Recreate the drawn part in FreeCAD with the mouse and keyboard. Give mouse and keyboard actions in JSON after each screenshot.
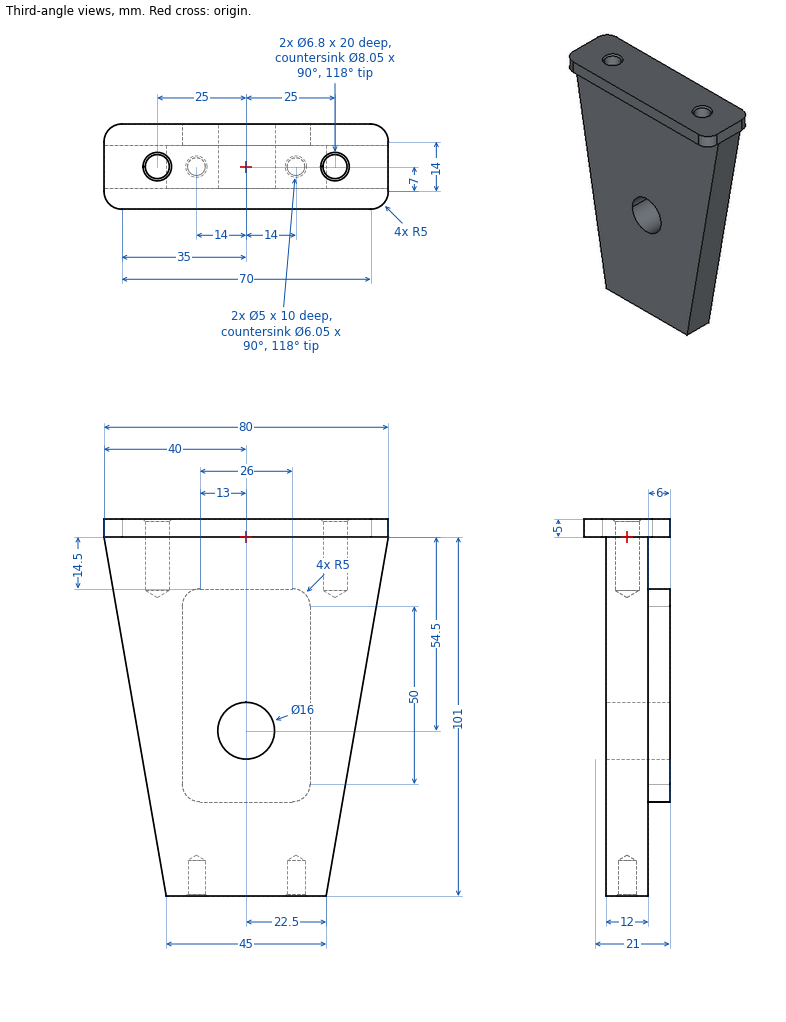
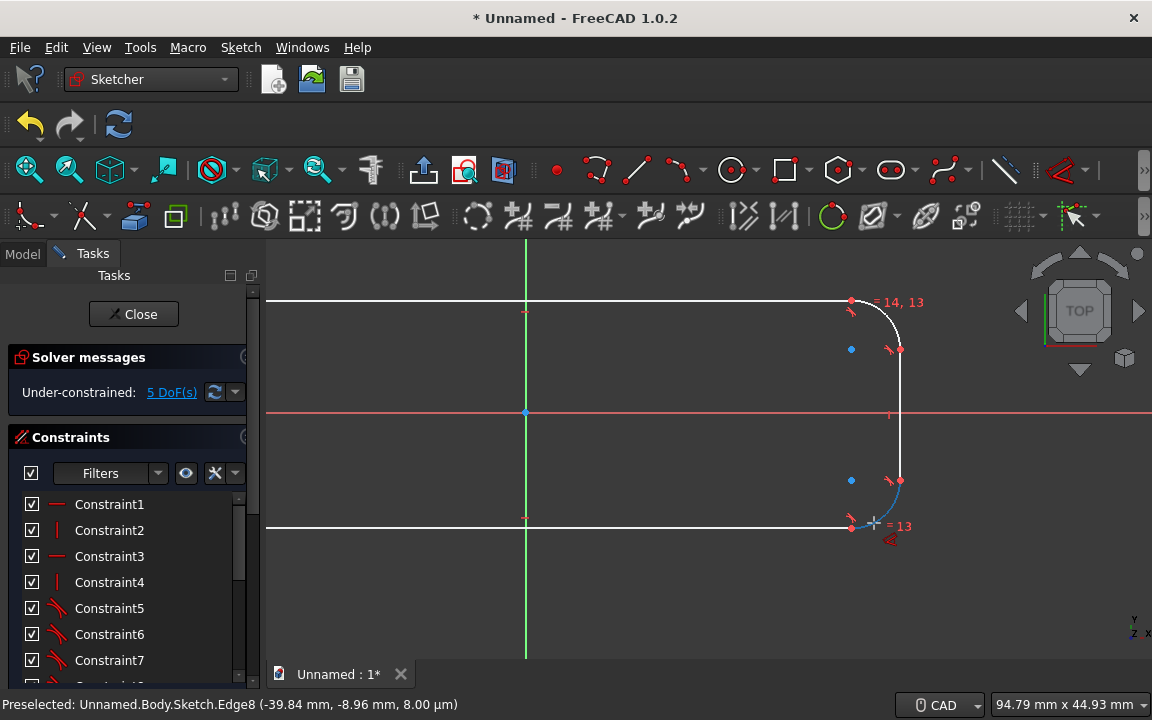
{"action": "left_click", "coordinate": [874, 523]}
{"action": "left_click", "coordinate": [889, 551]}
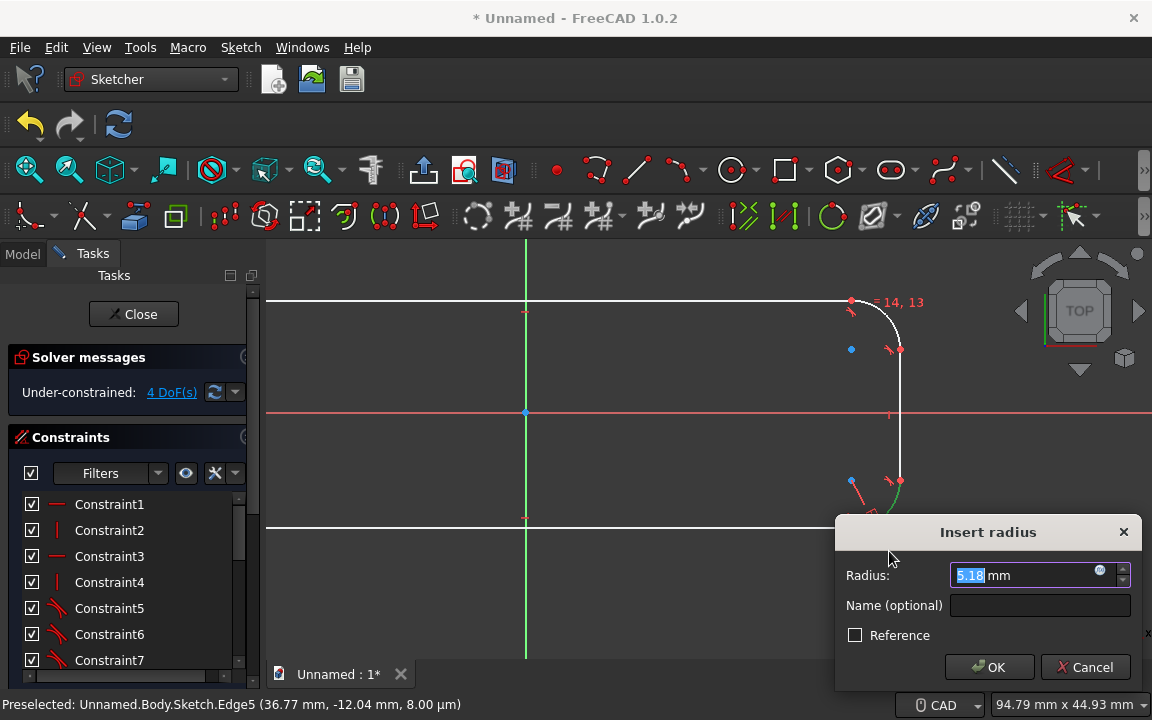
{"action": "type", "text": "5"}
{"action": "key", "text": "Return"}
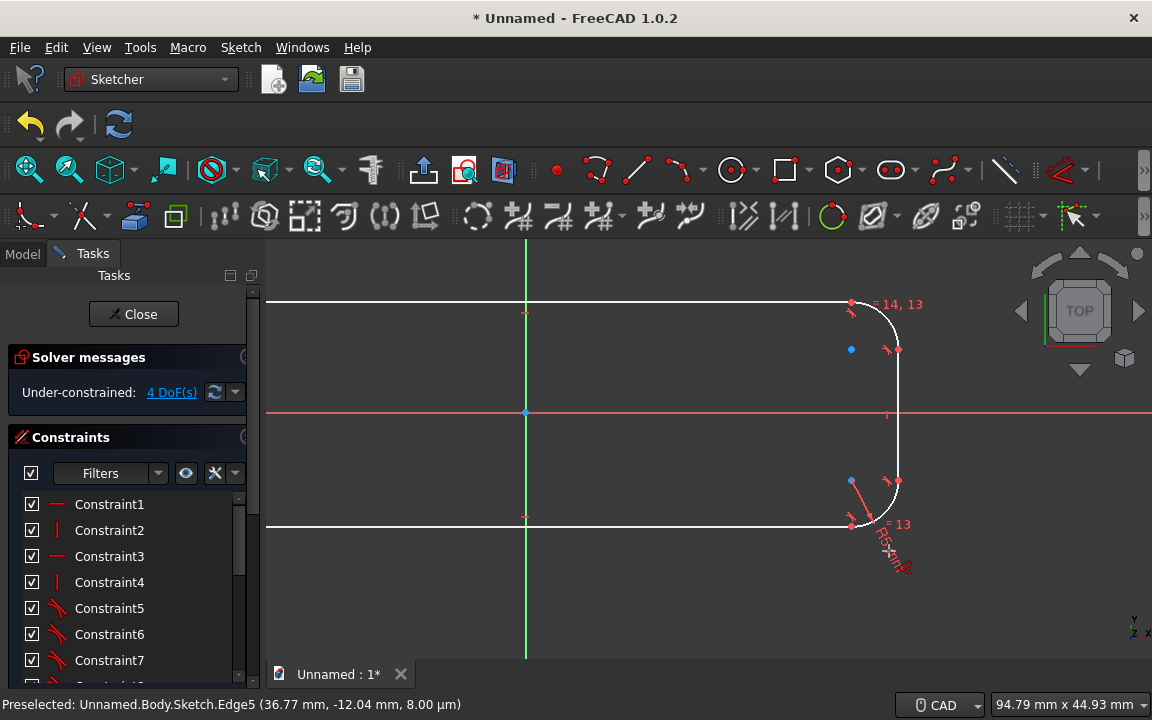
{"action": "left_click", "coordinate": [394, 527]}
{"action": "left_click", "coordinate": [573, 561]}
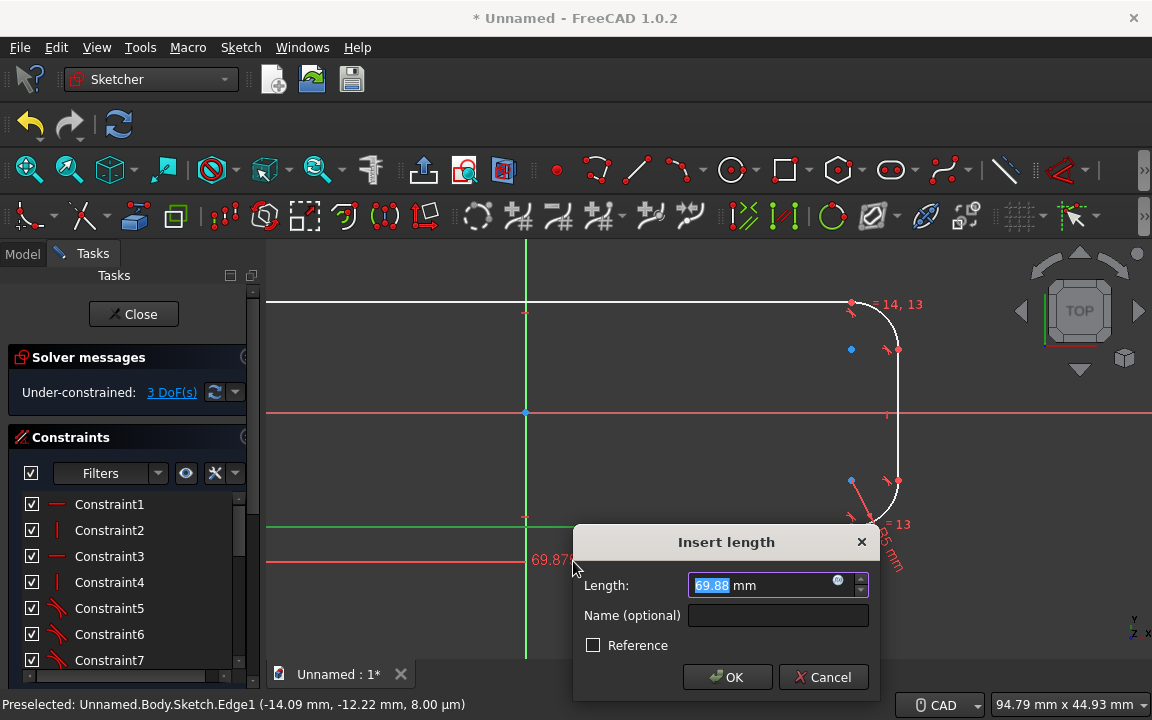
{"action": "type", "text": "70"}
{"action": "key", "text": "Return"}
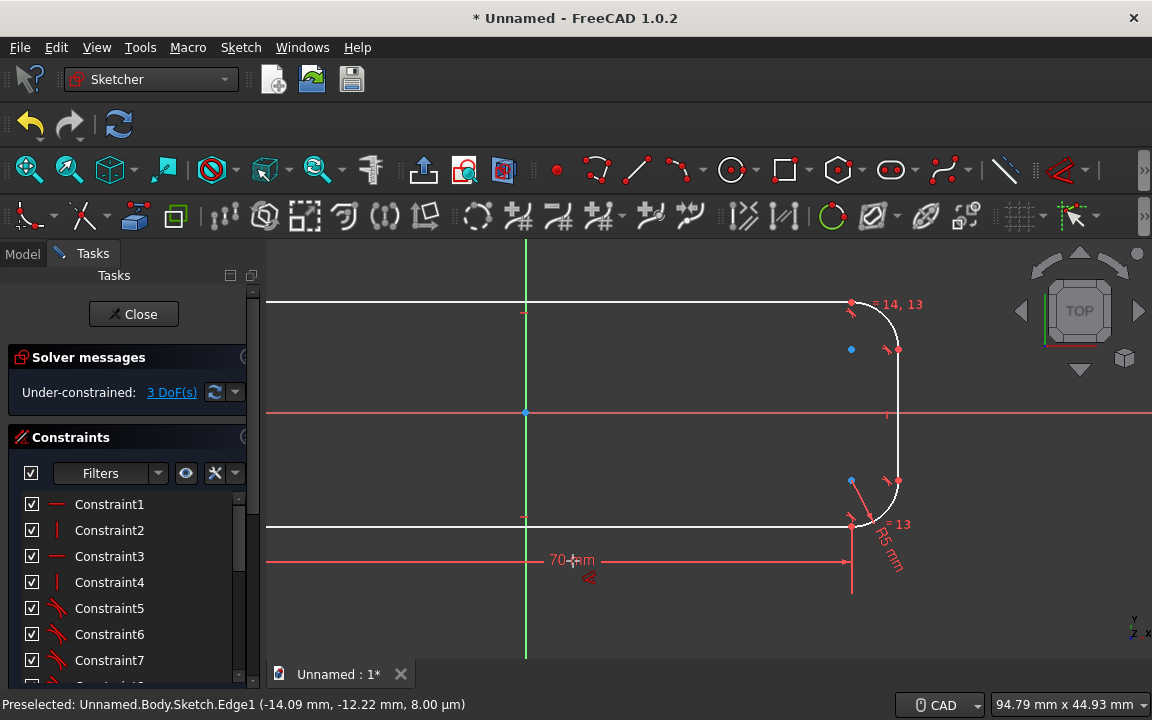
{"action": "left_click", "coordinate": [898, 441]}
{"action": "left_click", "coordinate": [932, 384]}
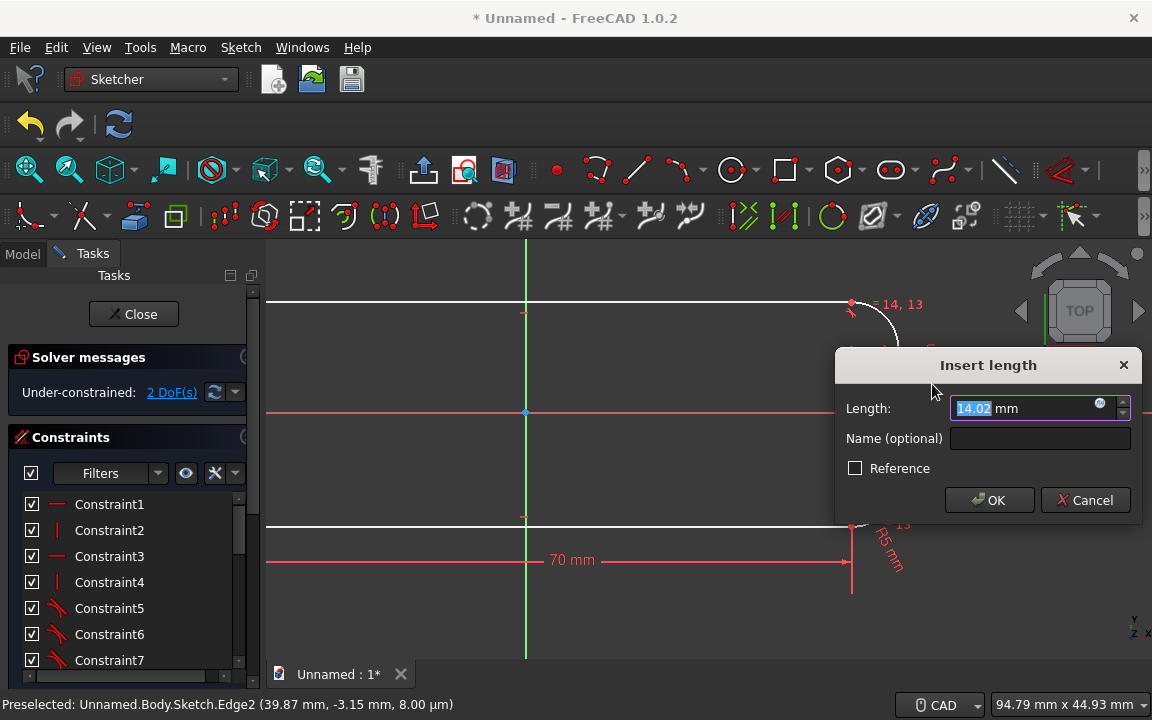
{"action": "type", "text": "14"}
{"action": "key", "text": "Return"}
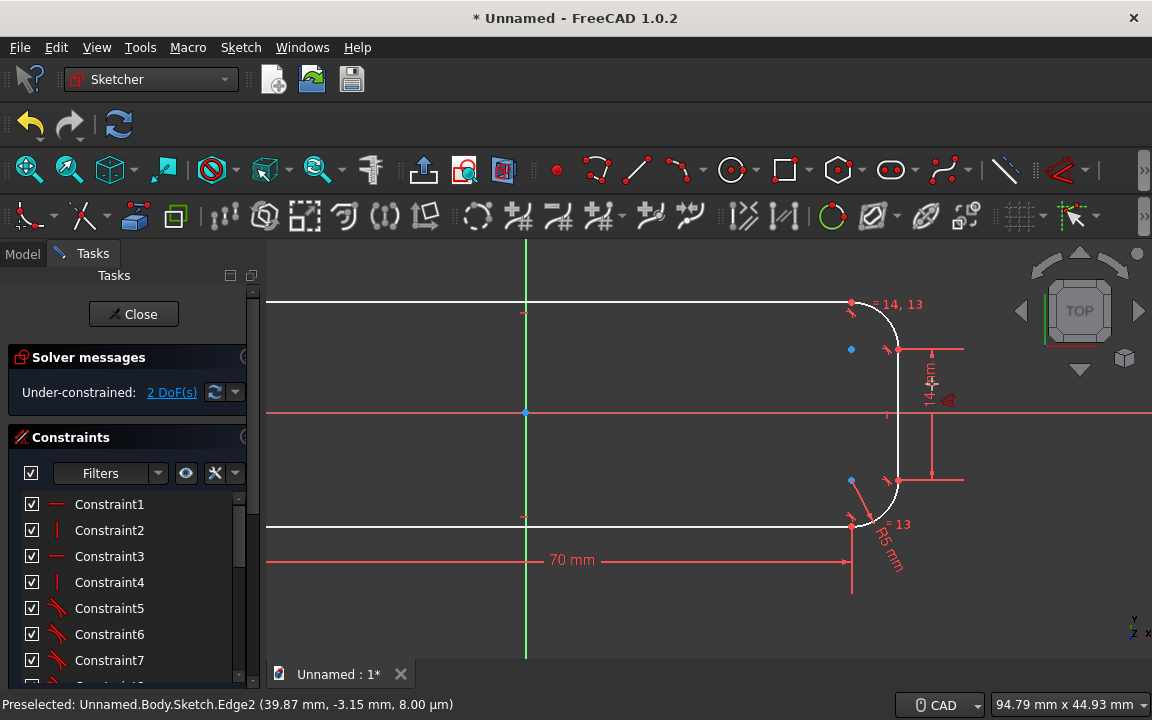
{"action": "left_click", "coordinate": [898, 480]}
{"action": "left_click", "coordinate": [932, 446]}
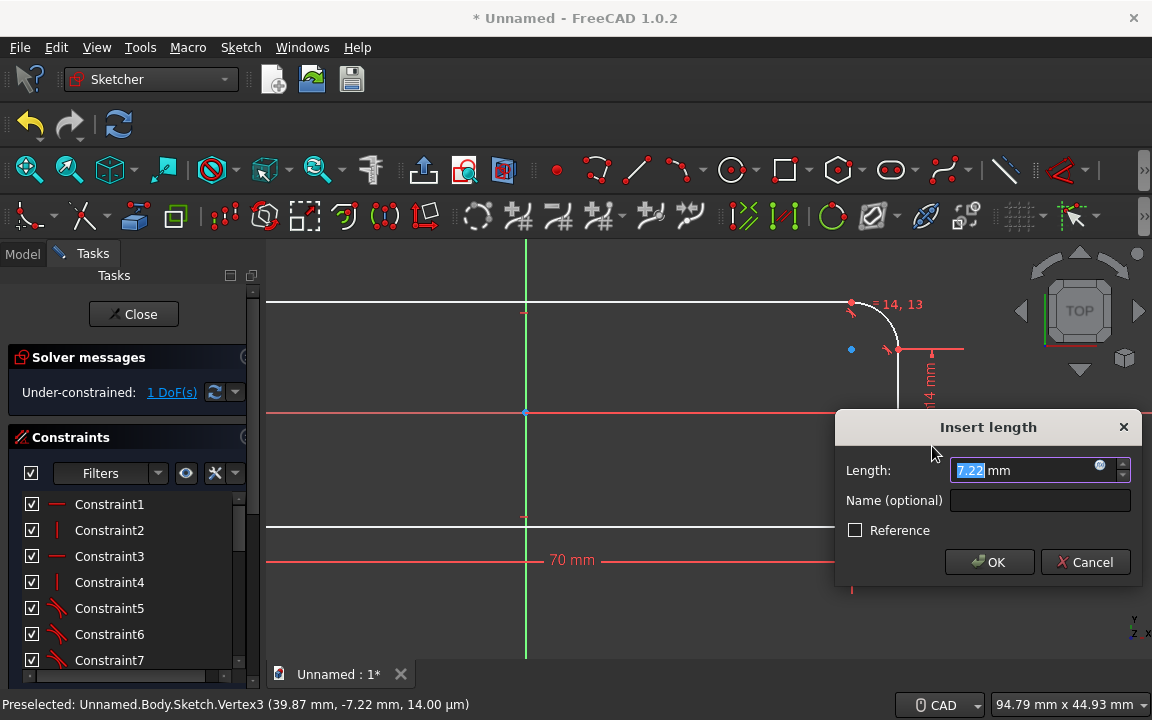
{"action": "type", "text": "7"}
{"action": "key", "text": "Return"}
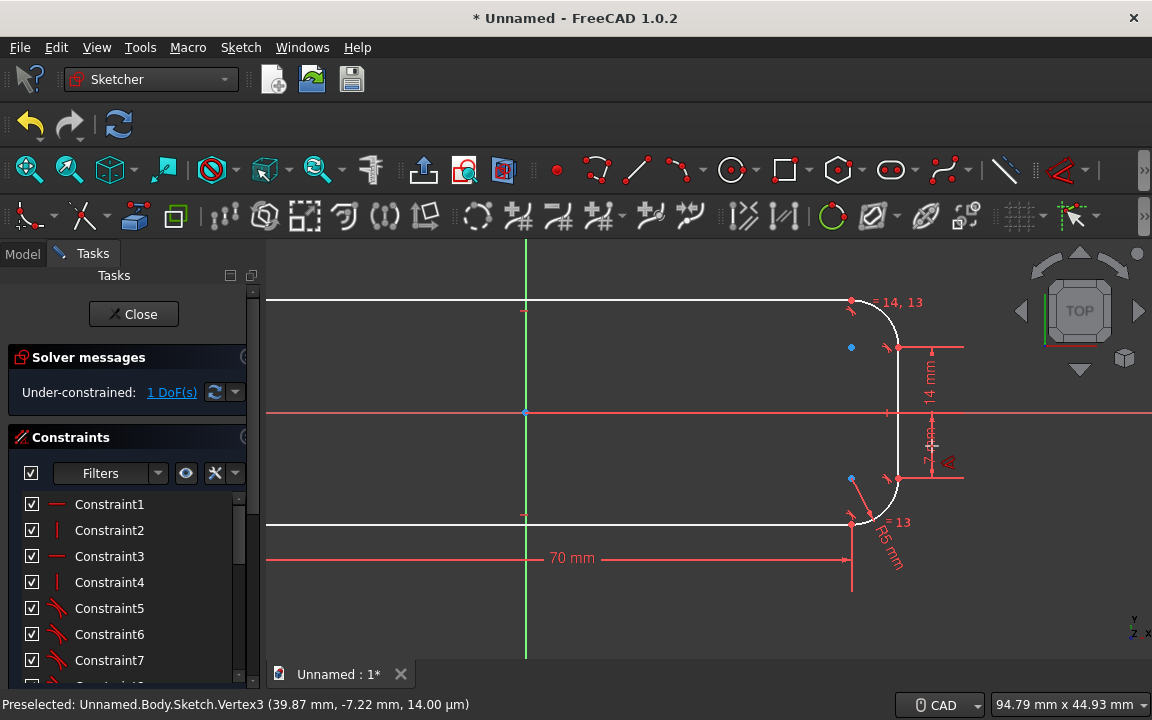
{"action": "scroll", "coordinate": [874, 523], "scroll_direction": "down", "scroll_amount": 2}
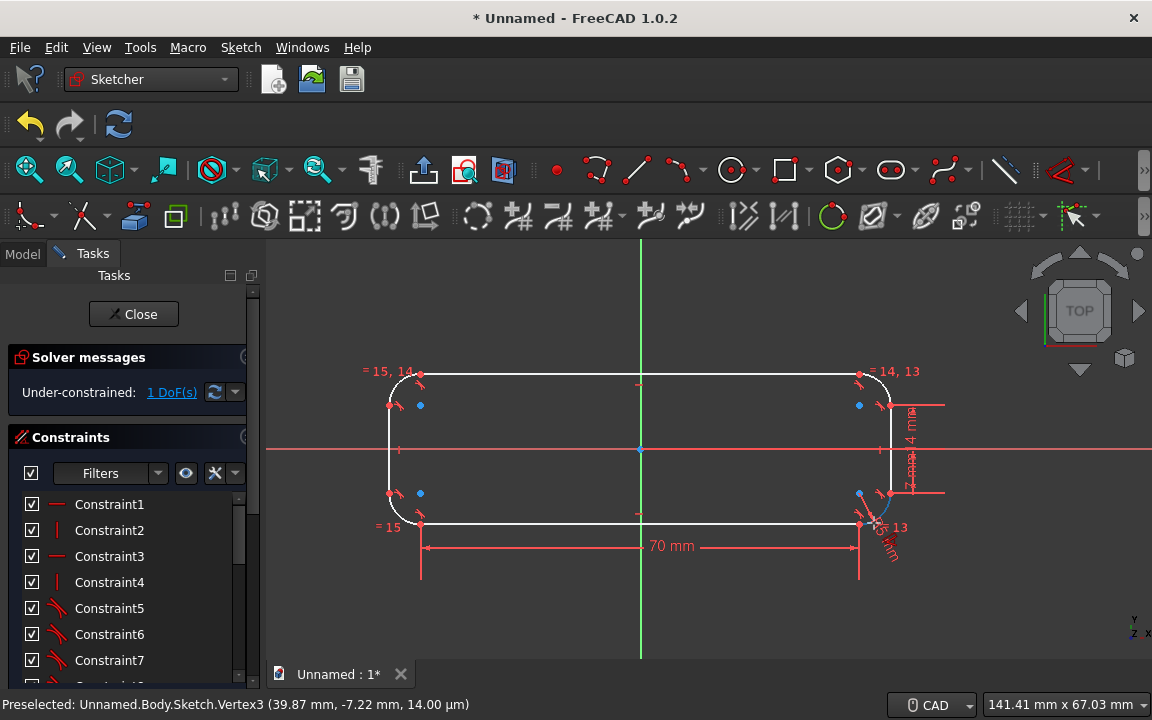
{"action": "left_click", "coordinate": [421, 524]}
{"action": "left_click", "coordinate": [531, 558]}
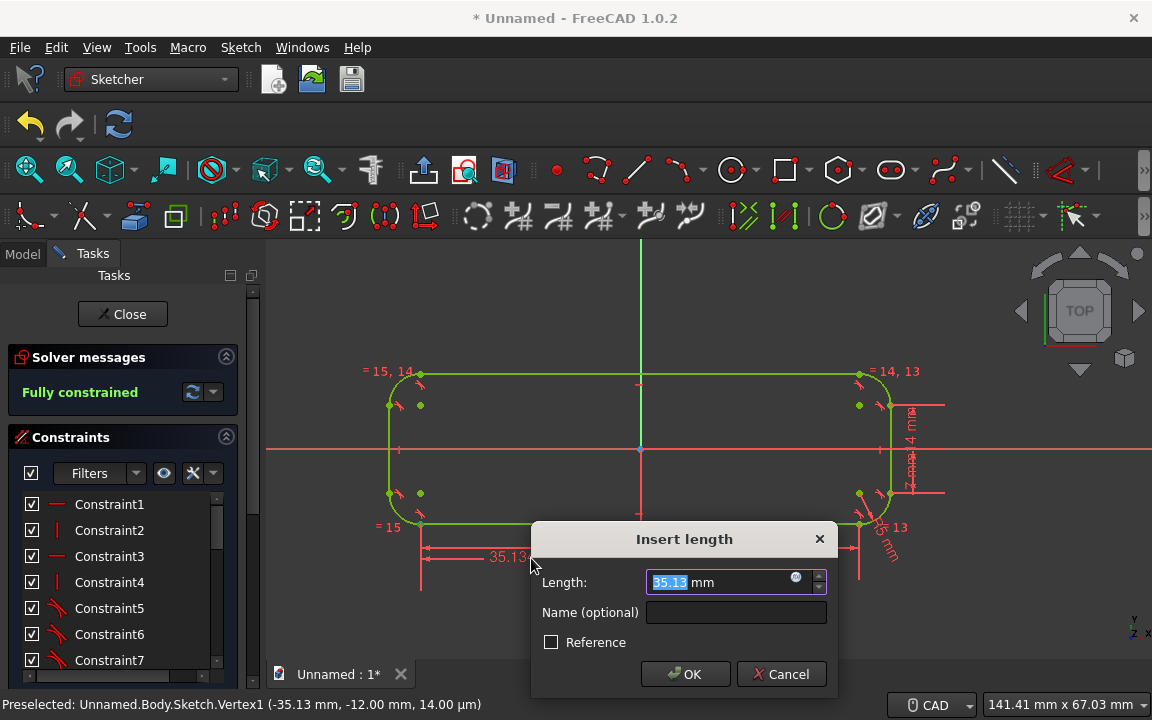
{"action": "type", "text": "35"}
{"action": "key", "text": "Return"}
{"action": "key", "text": "Escape"}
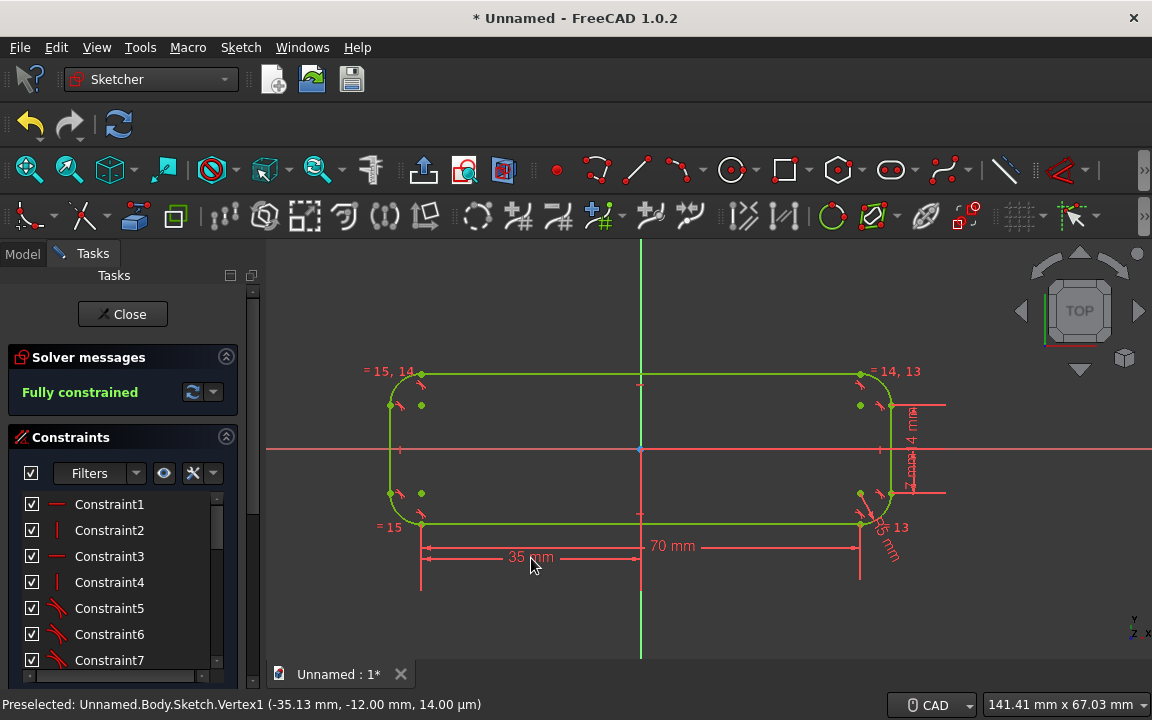
{"action": "left_click", "coordinate": [123, 314]}